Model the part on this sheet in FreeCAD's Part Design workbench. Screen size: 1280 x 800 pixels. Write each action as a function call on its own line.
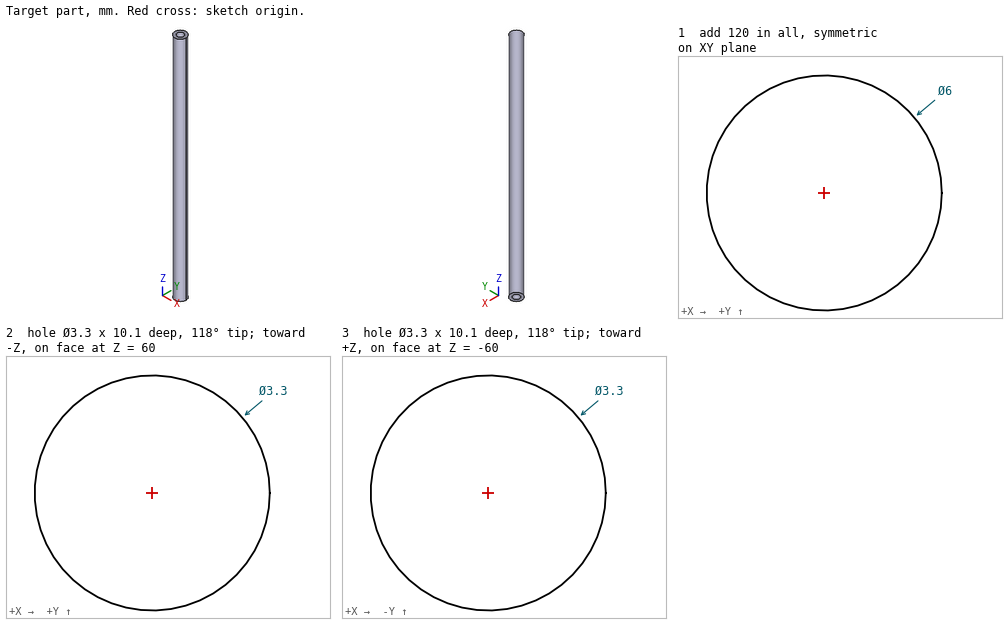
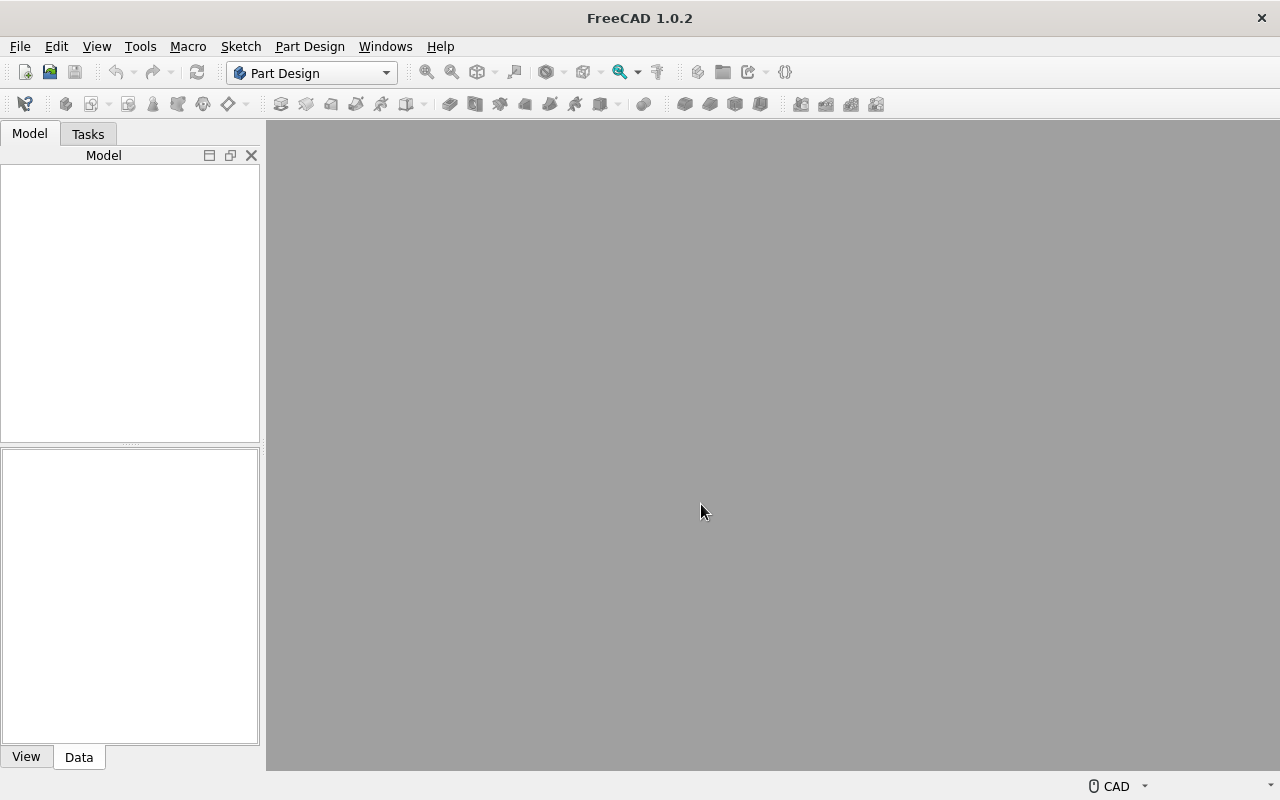
click(25, 72)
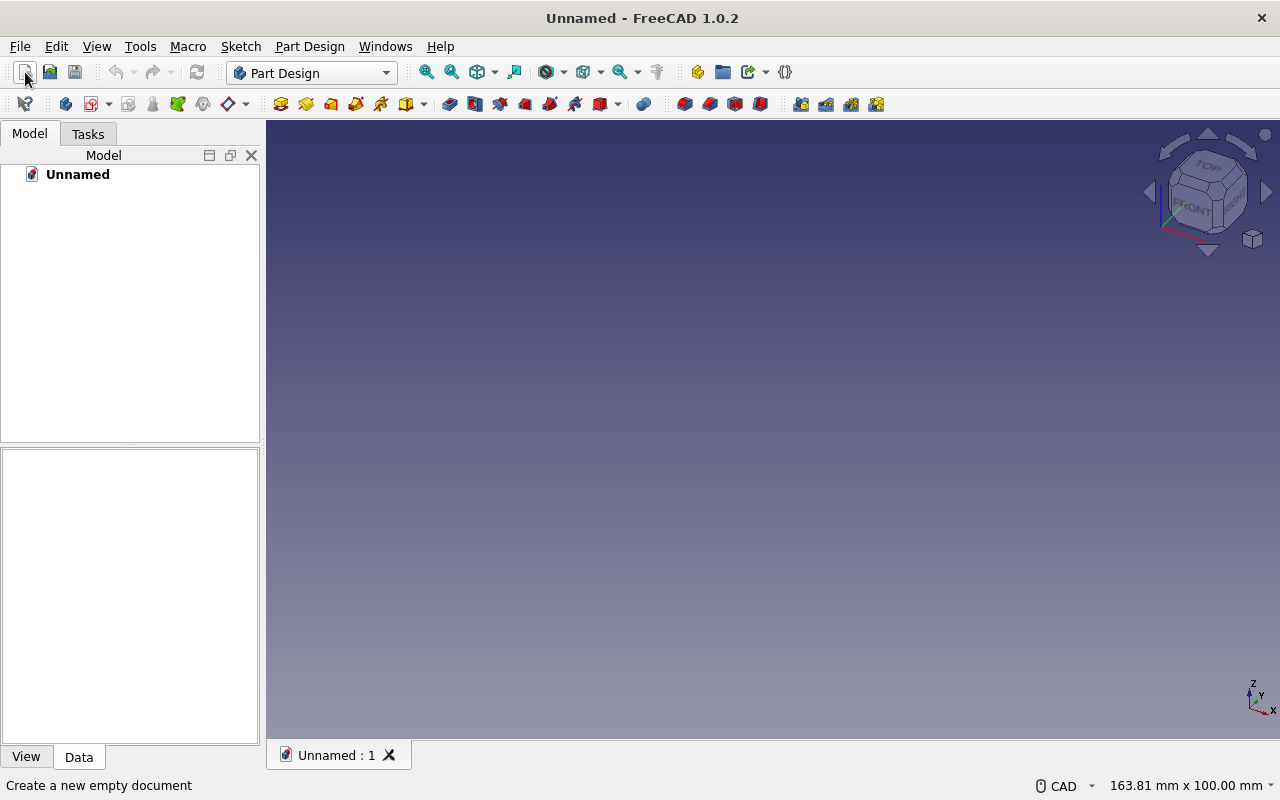
click(90, 104)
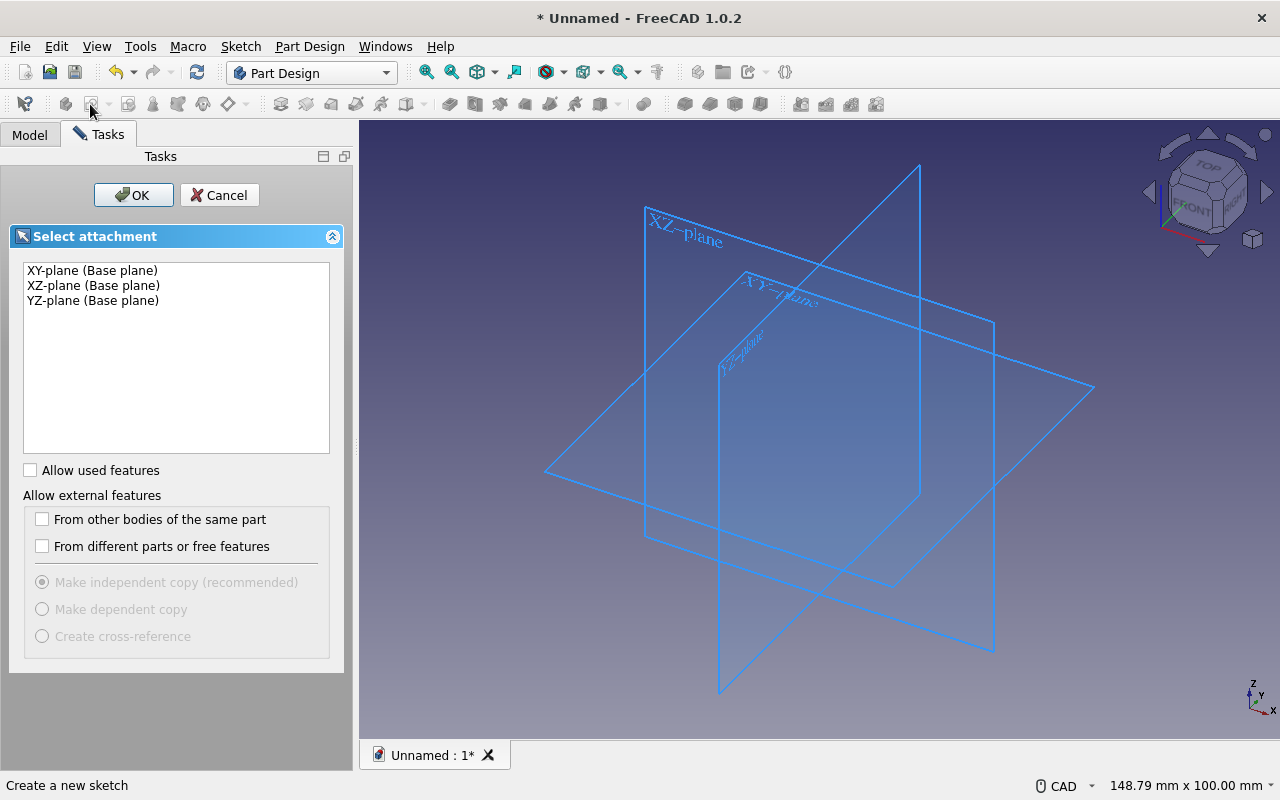
click(84, 270)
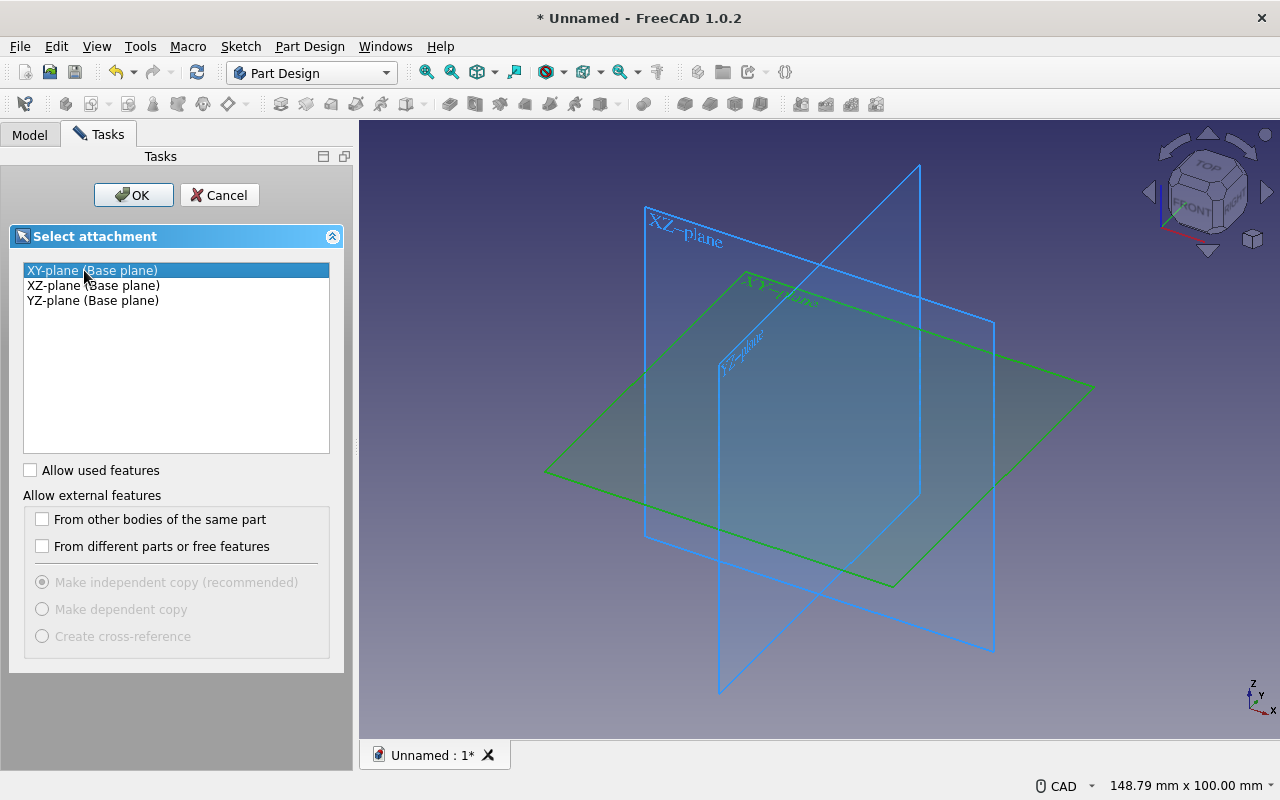
click(134, 195)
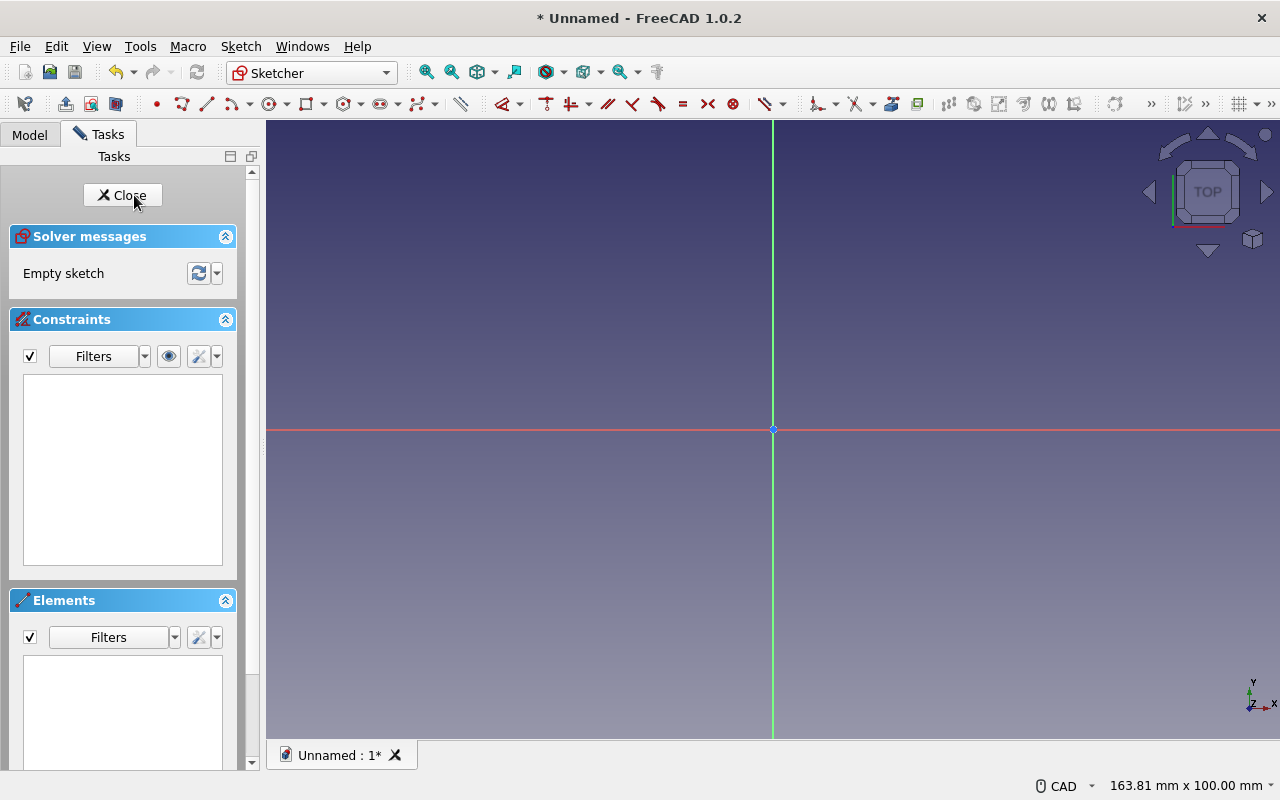
scroll(780, 429, up, 12)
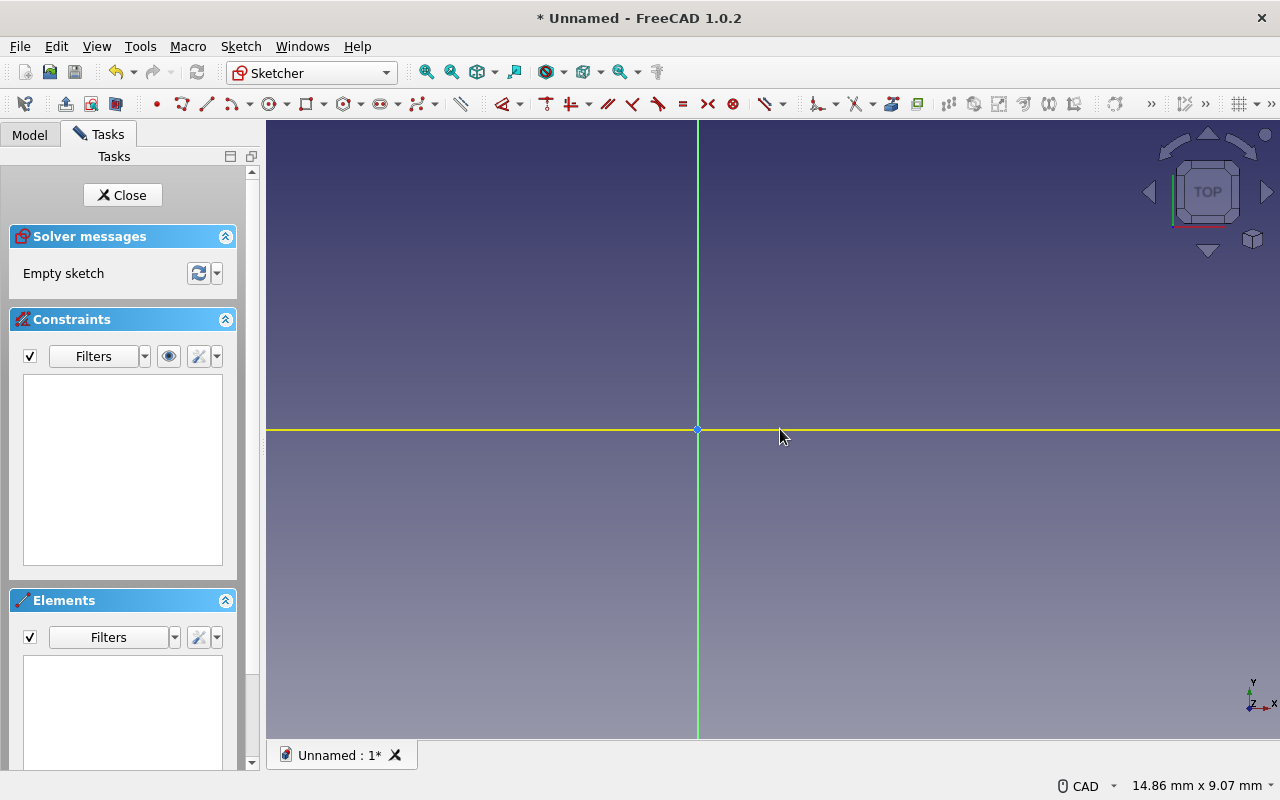
click(268, 104)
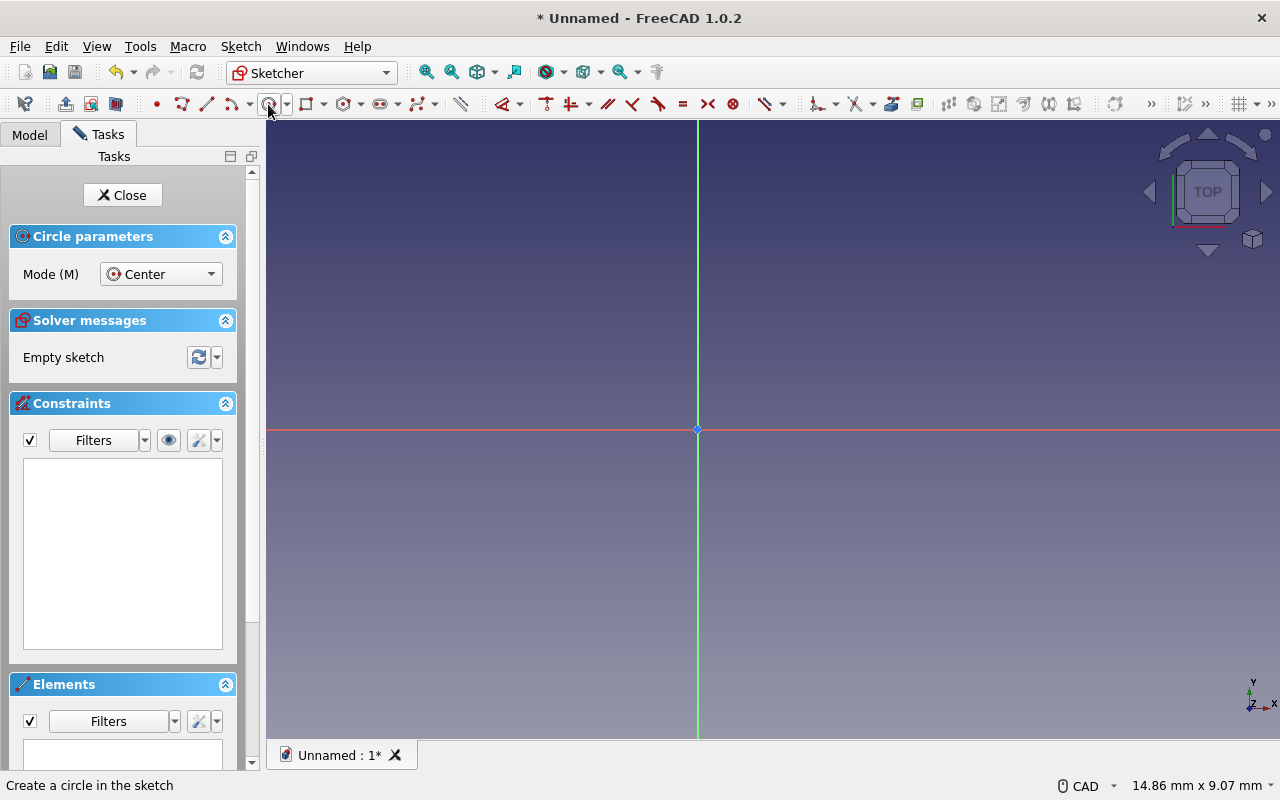
click(698, 430)
click(842, 285)
key(Escape)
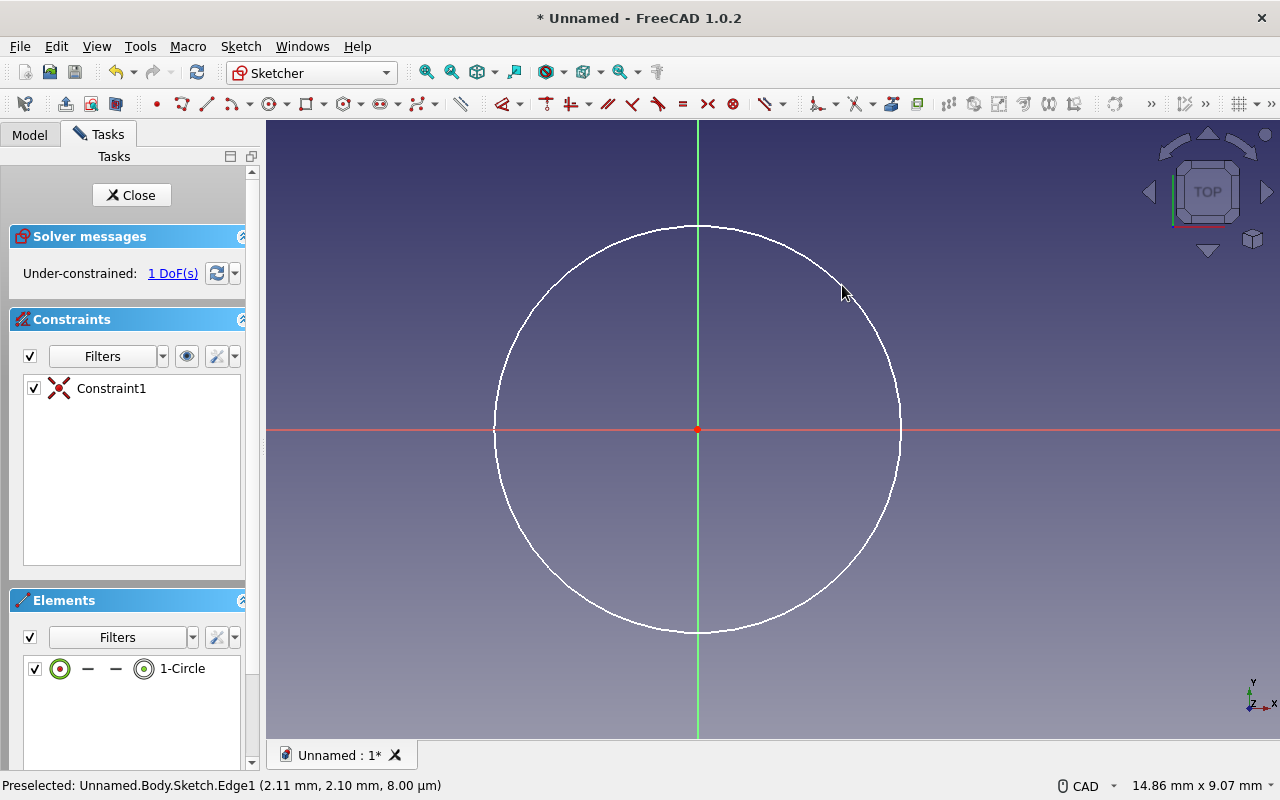
click(502, 104)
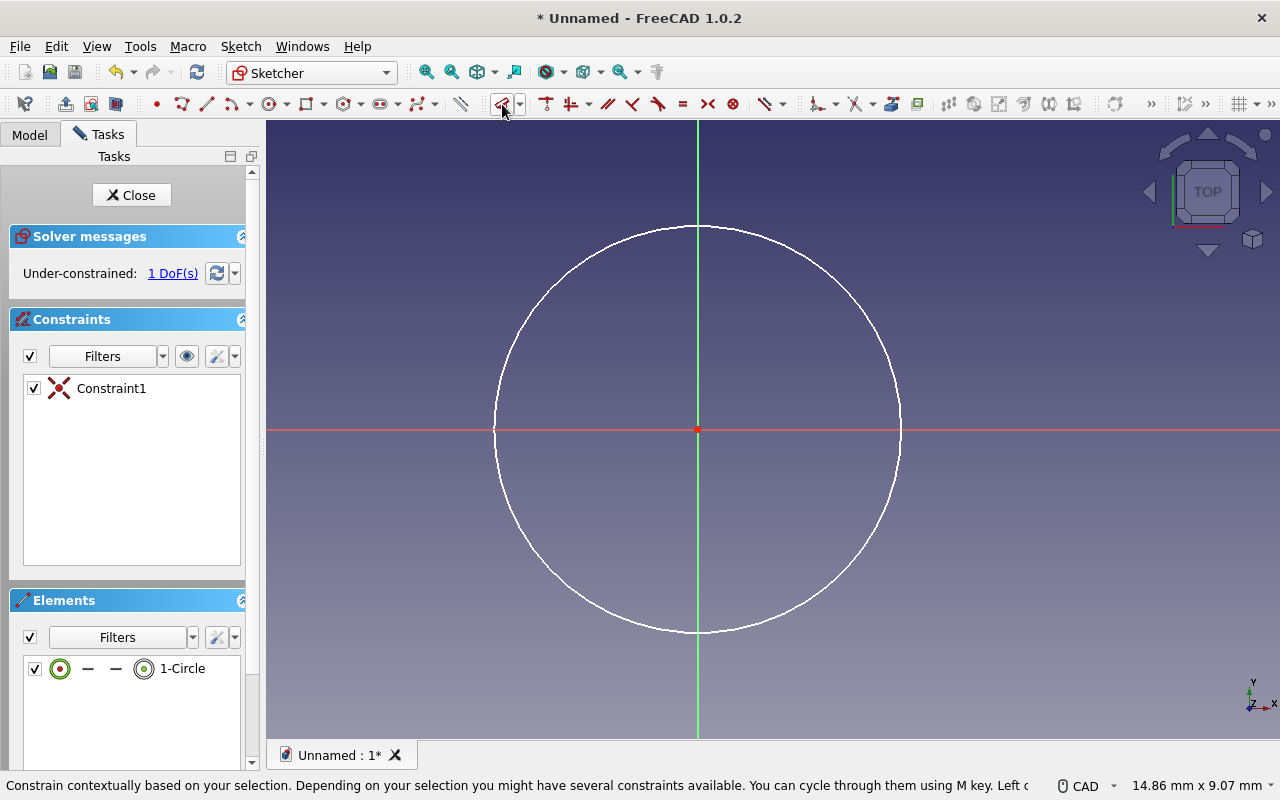
click(841, 285)
click(864, 262)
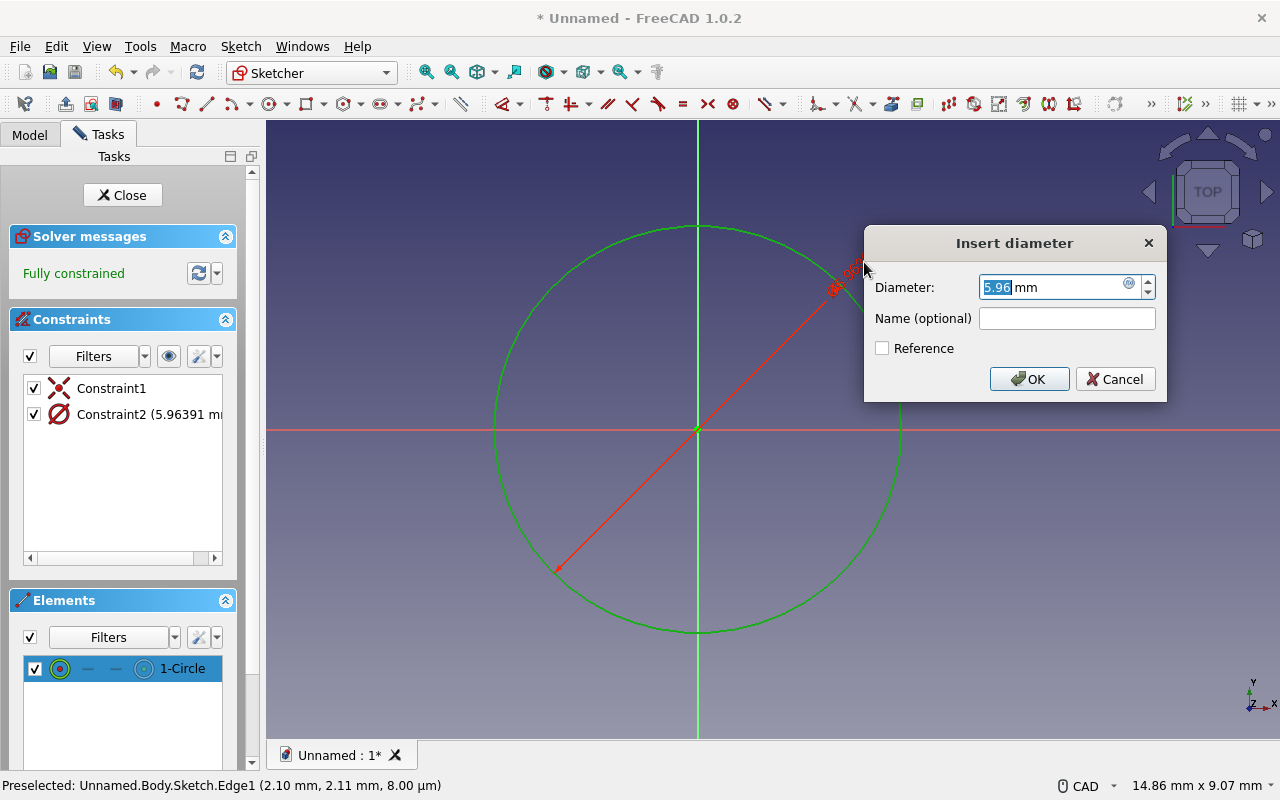
text(6)
key(Return)
key(Escape)